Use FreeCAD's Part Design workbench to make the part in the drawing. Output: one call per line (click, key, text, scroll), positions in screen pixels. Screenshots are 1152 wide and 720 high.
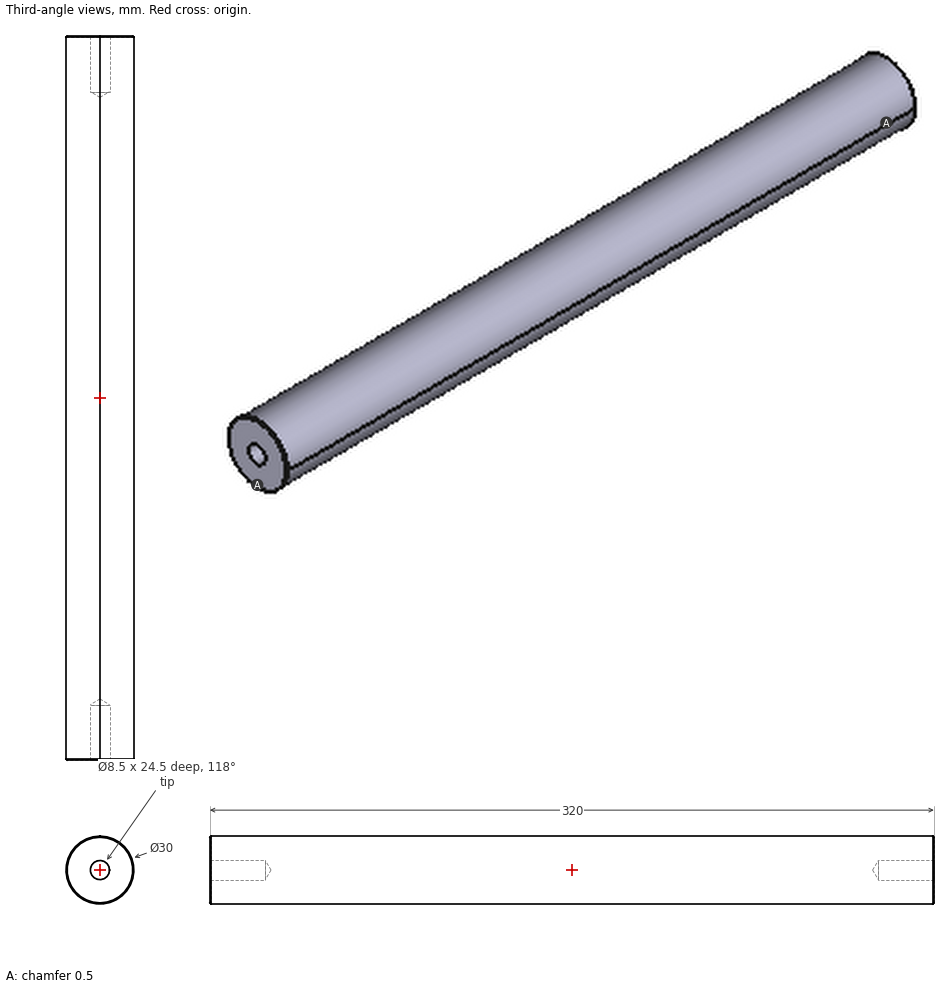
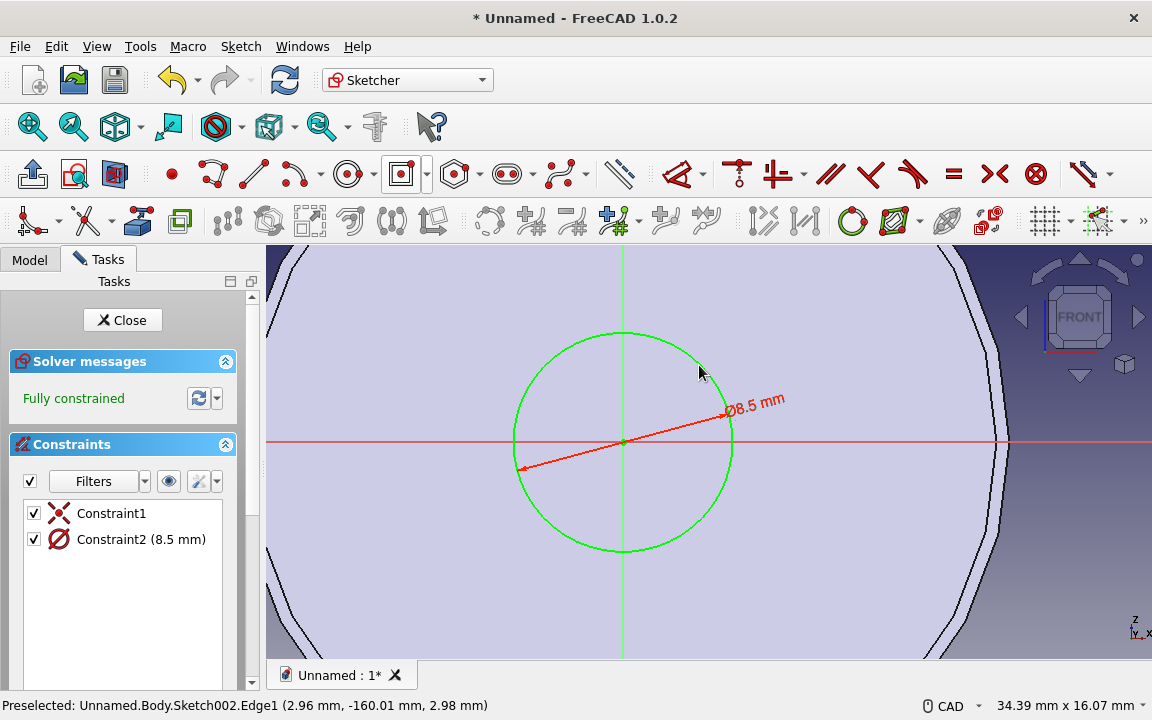
click(123, 320)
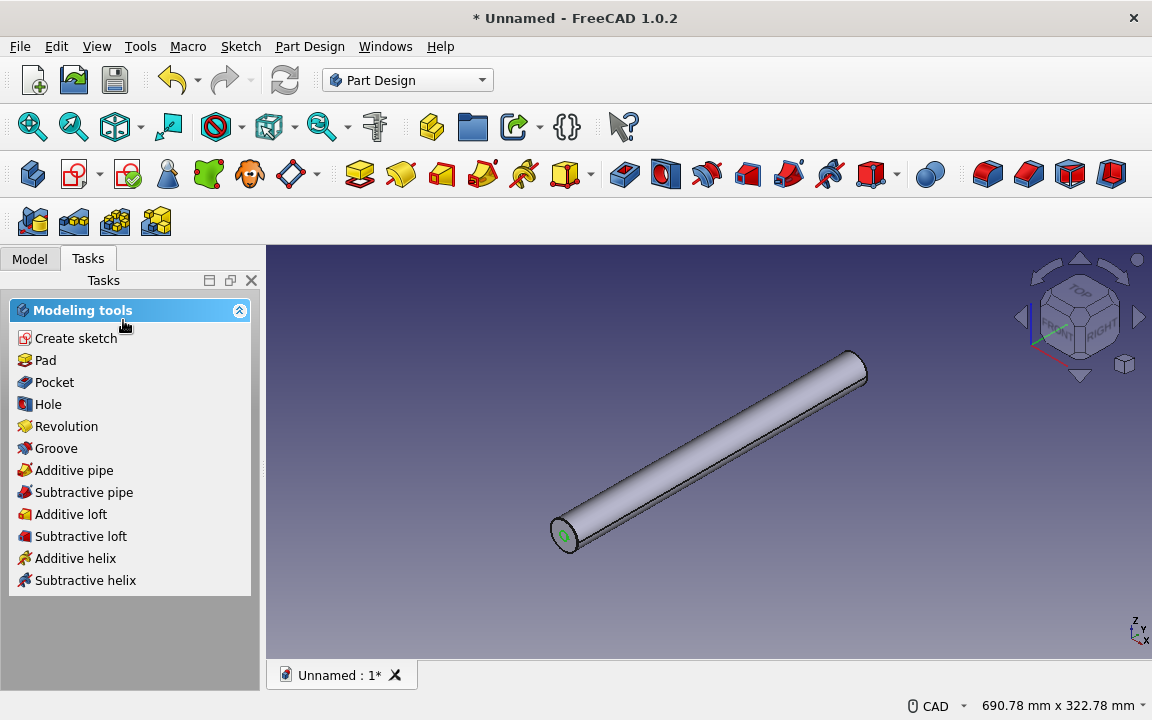
click(666, 174)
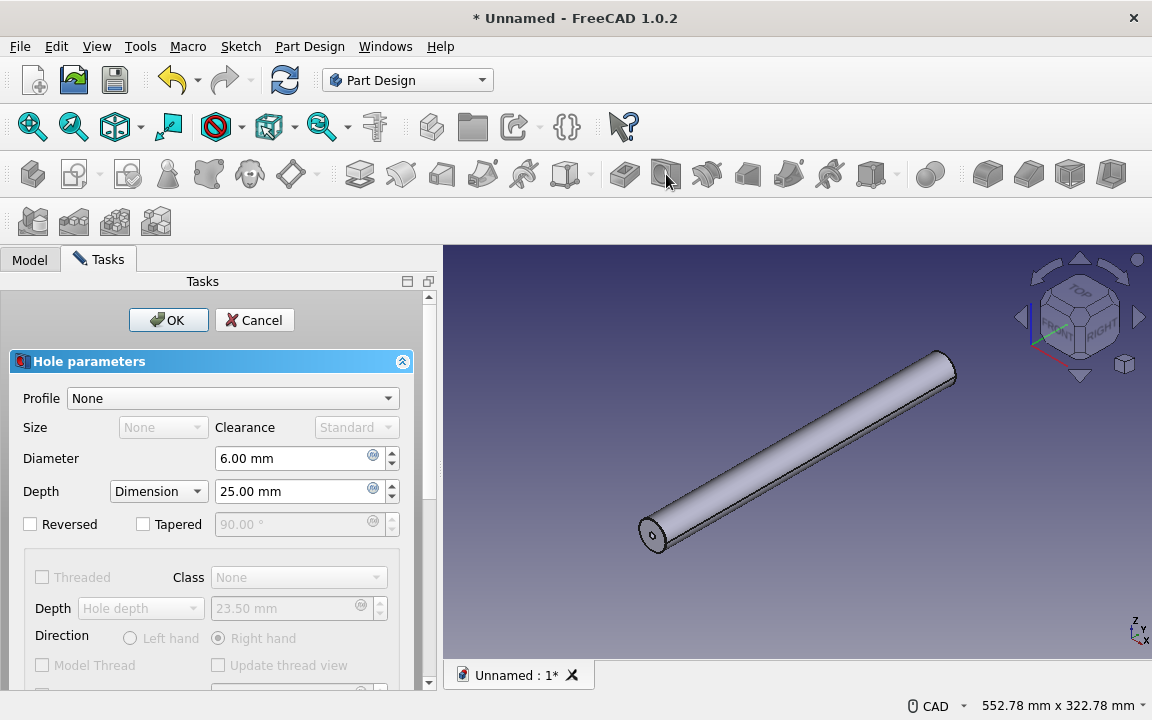
triple_click(300, 458)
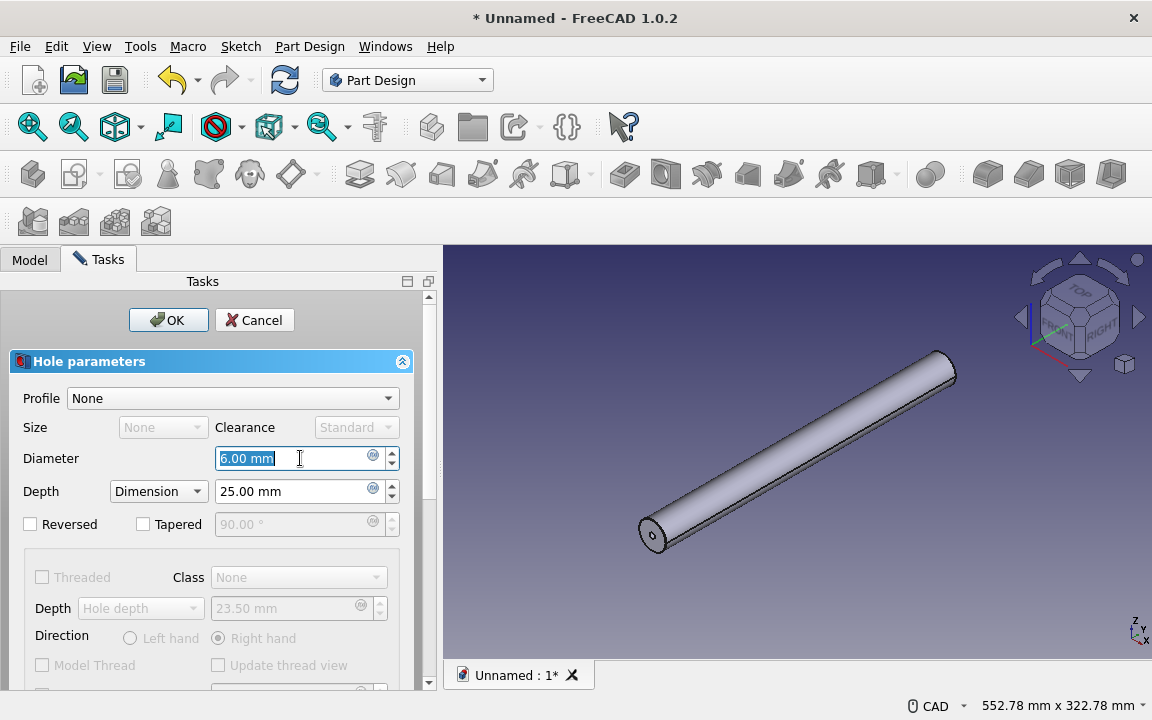
text(8.5)
key(Tab)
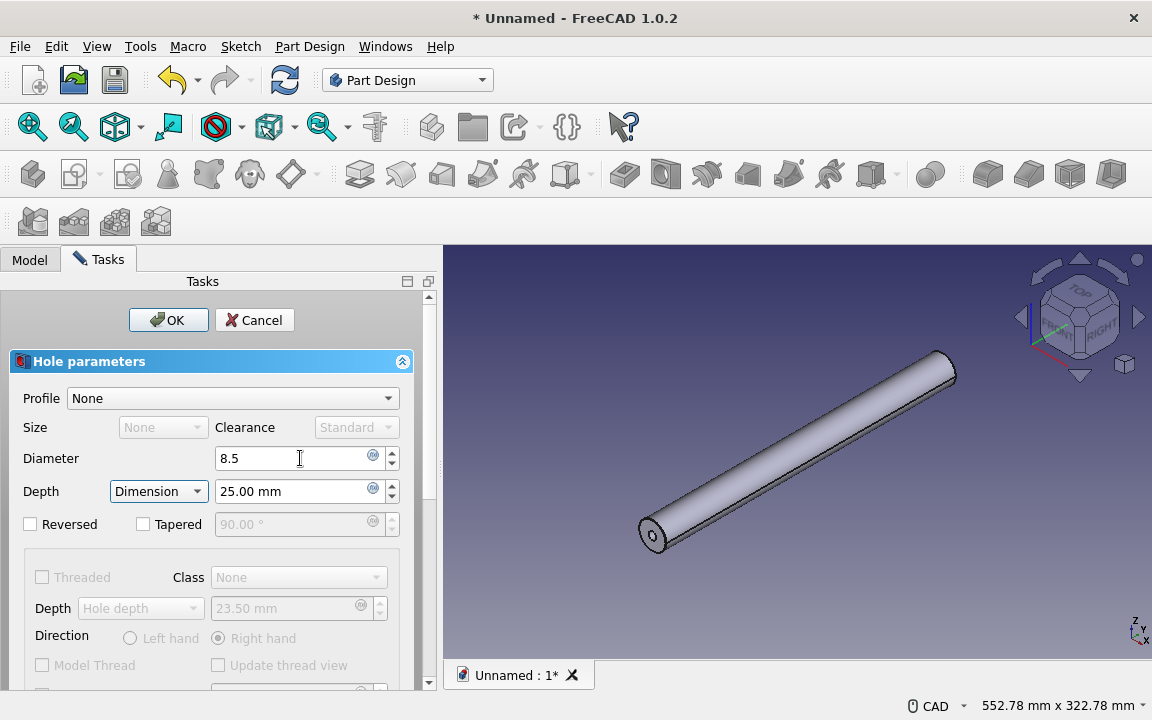
triple_click(300, 492)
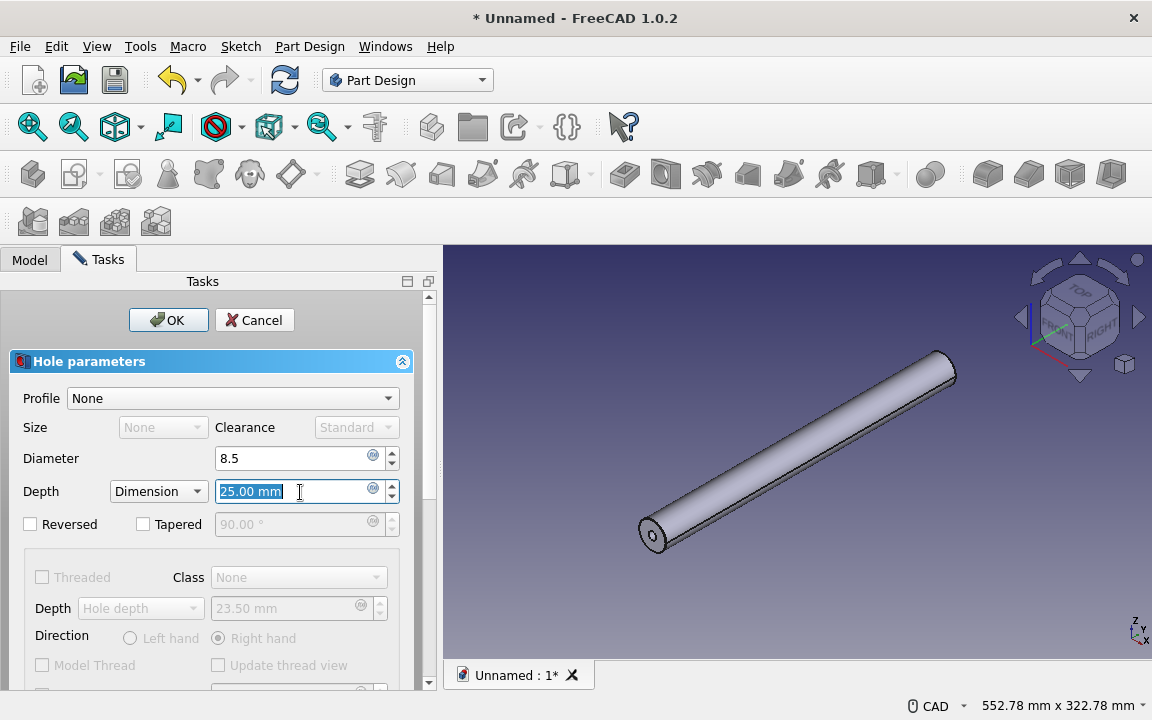
text(24.5)
key(Tab)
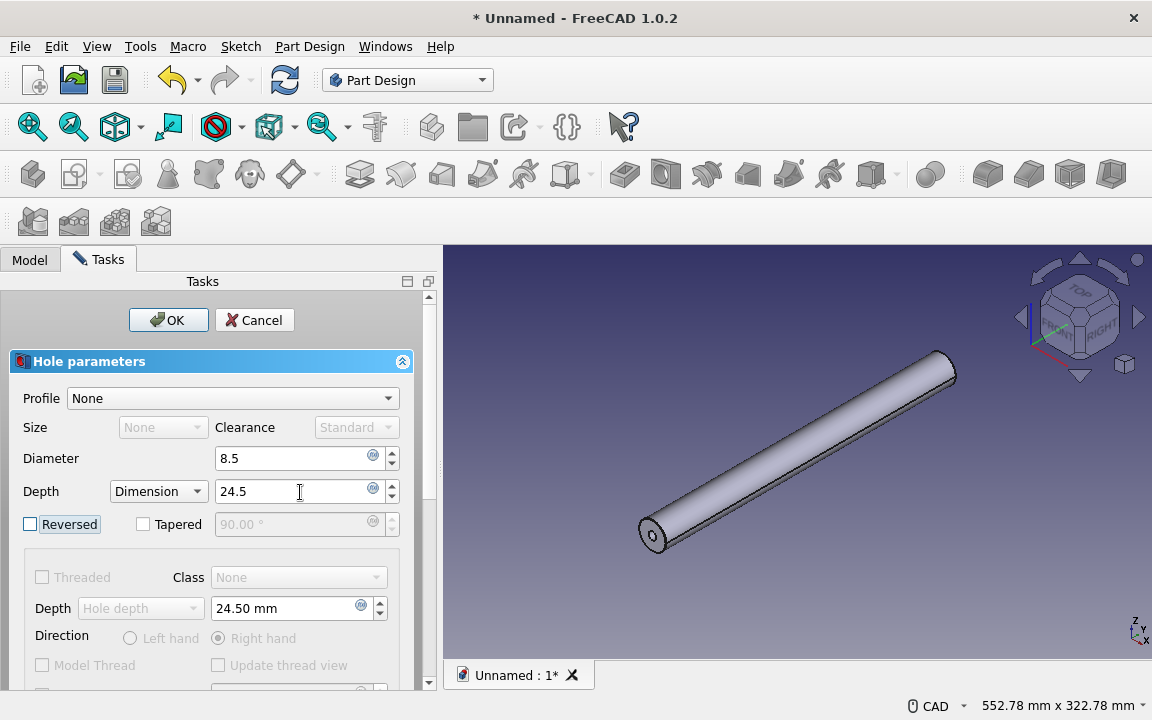
click(169, 320)